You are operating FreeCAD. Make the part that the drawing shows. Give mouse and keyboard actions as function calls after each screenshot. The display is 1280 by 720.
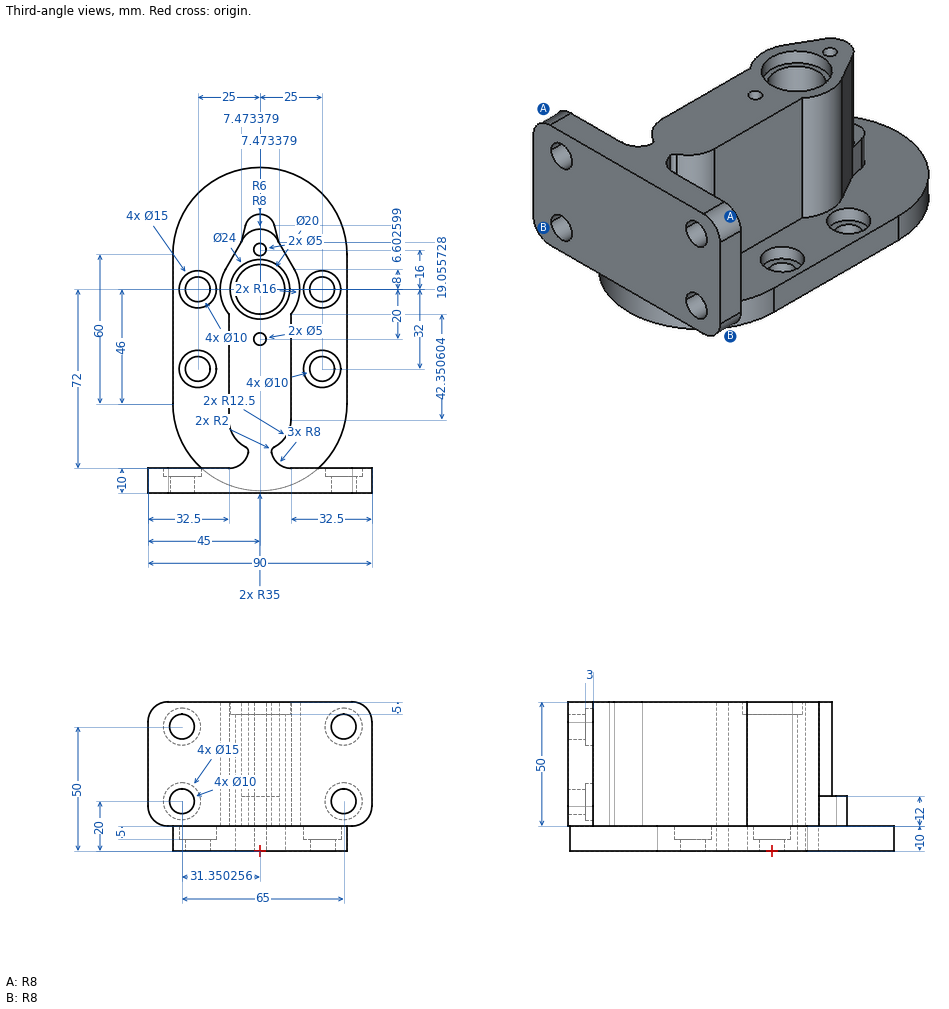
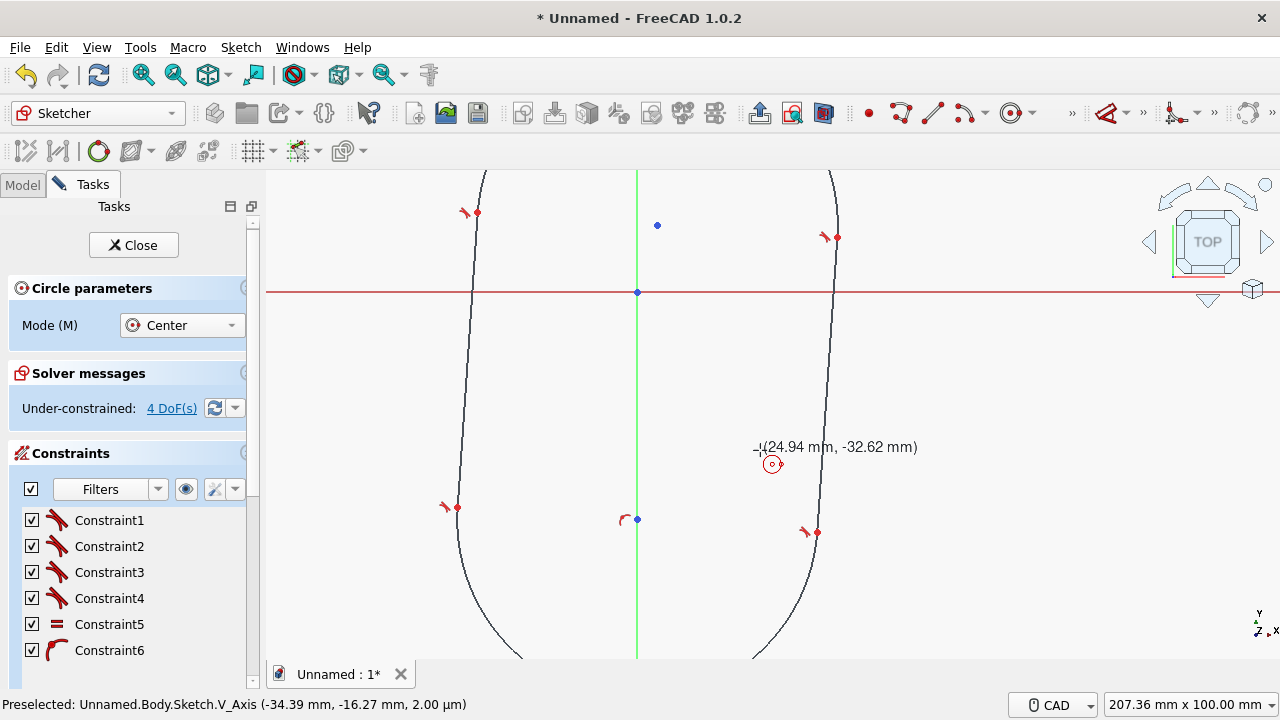
click(760, 448)
click(777, 431)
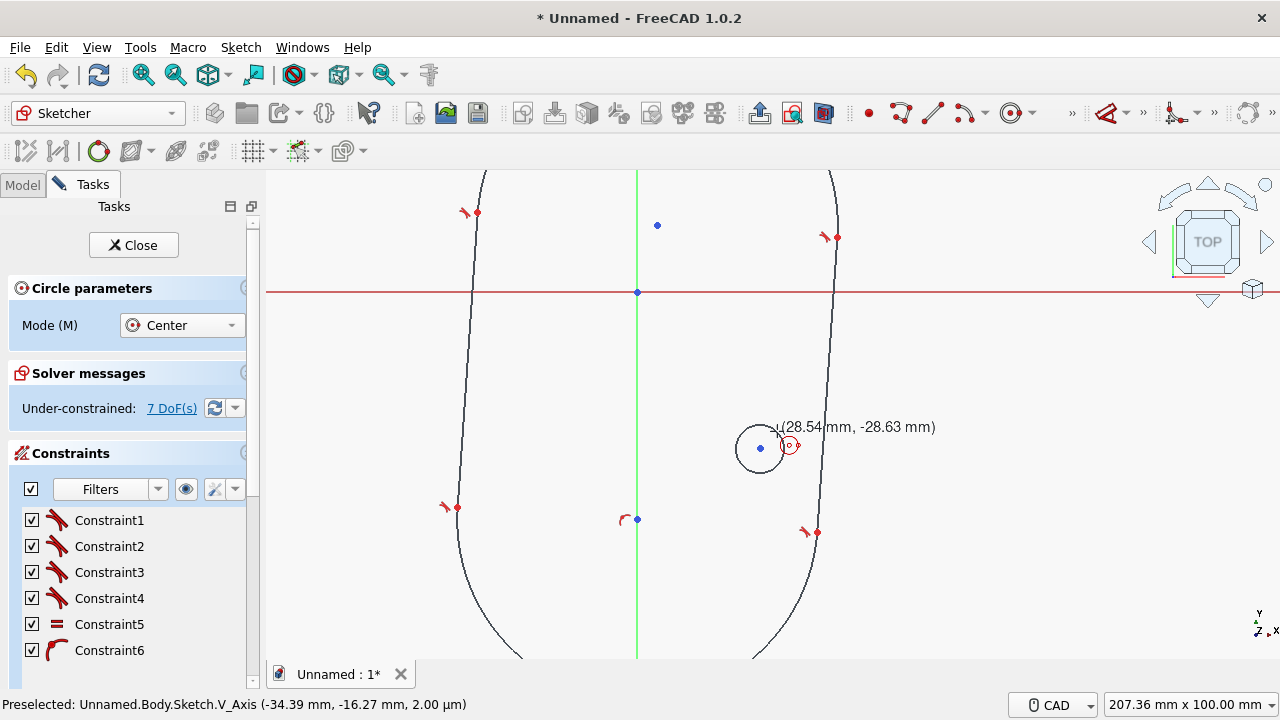
click(515, 448)
click(532, 431)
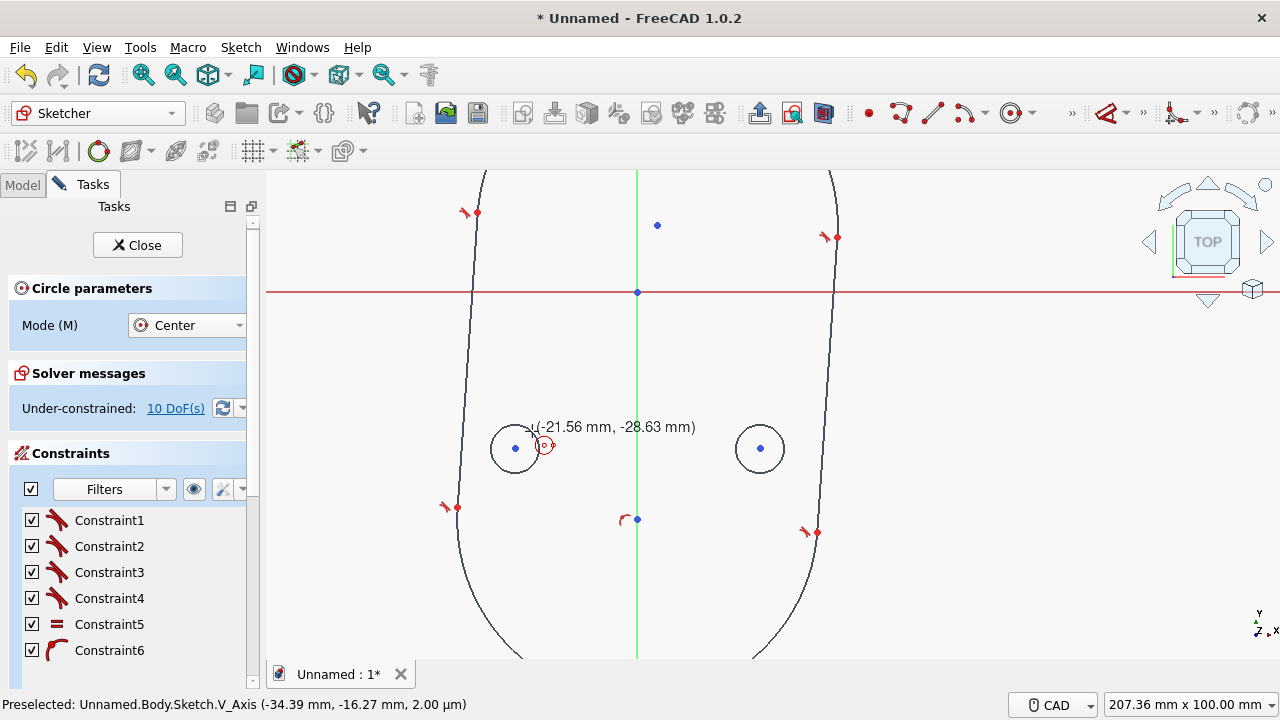
click(760, 292)
click(777, 275)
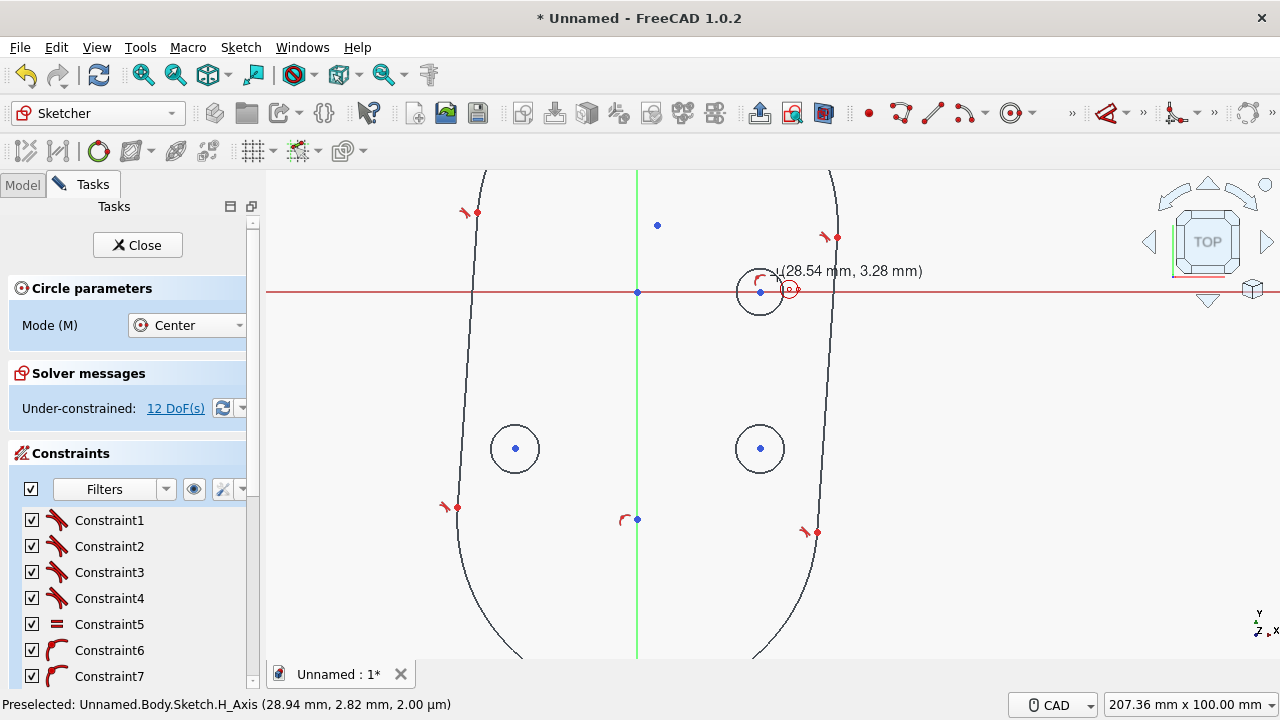
click(515, 292)
click(532, 275)
key(Escape)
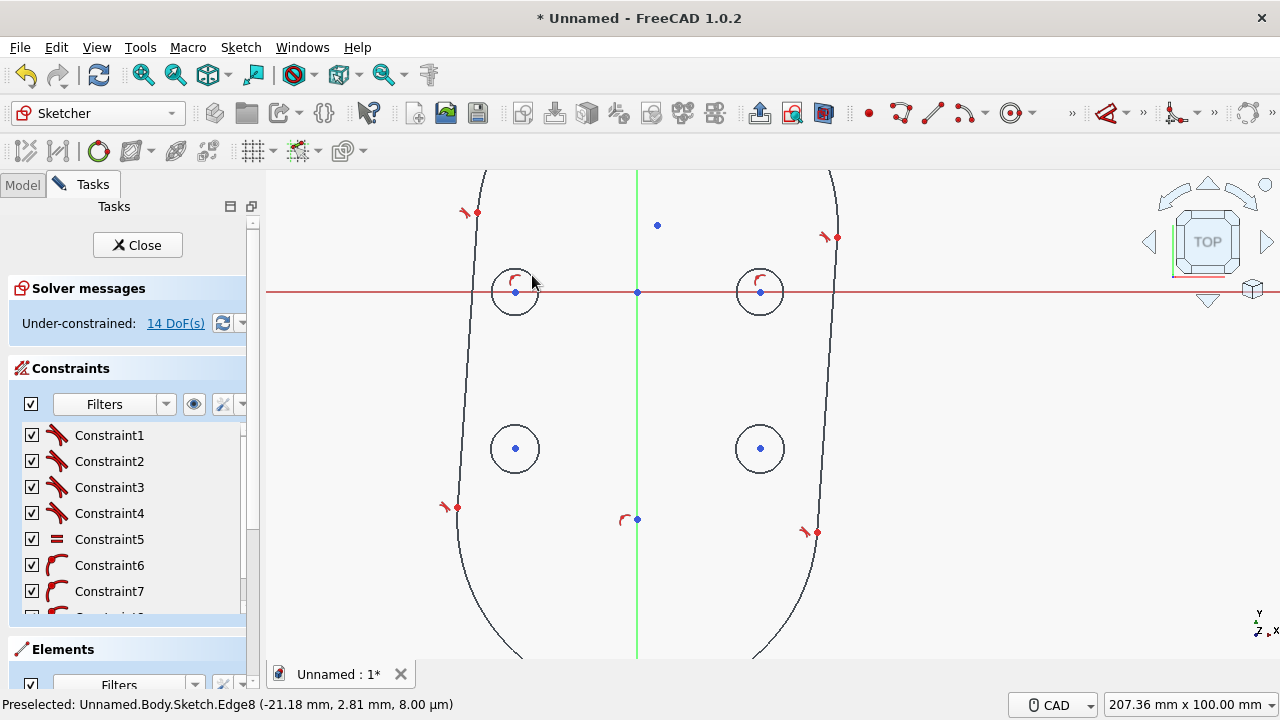
click(464, 419)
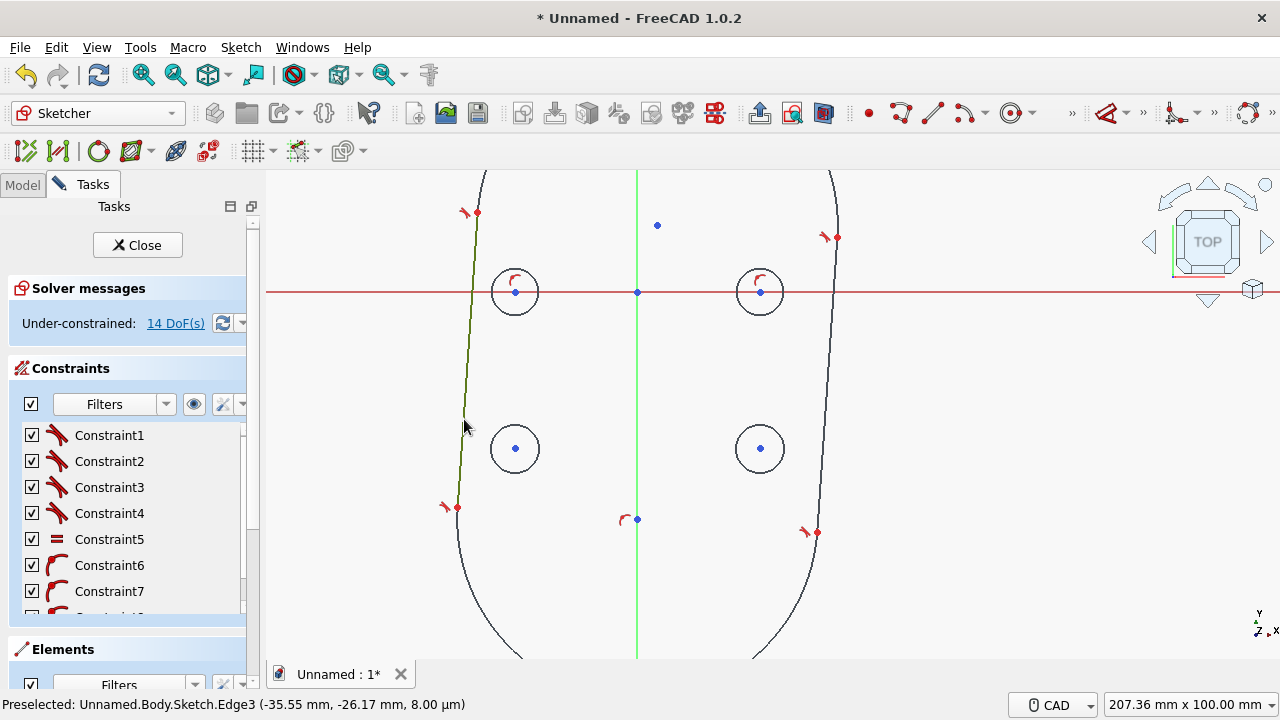
key(v)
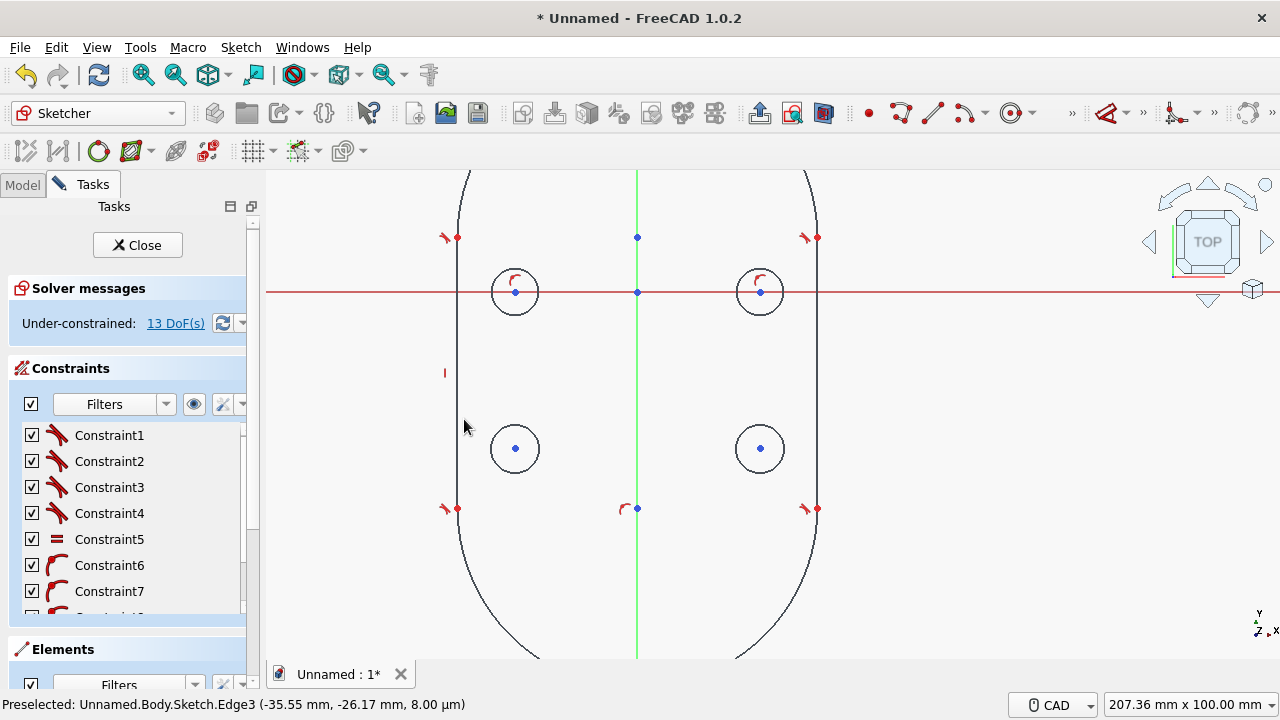
click(777, 432)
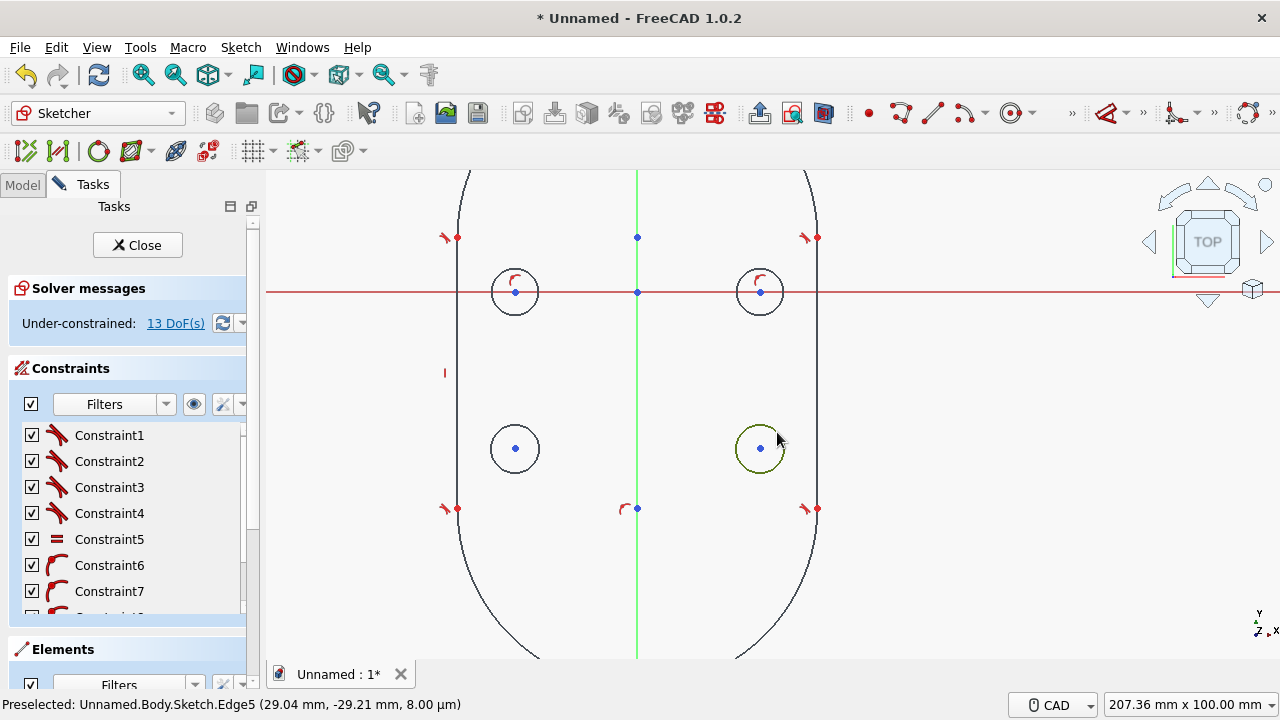
click(532, 432)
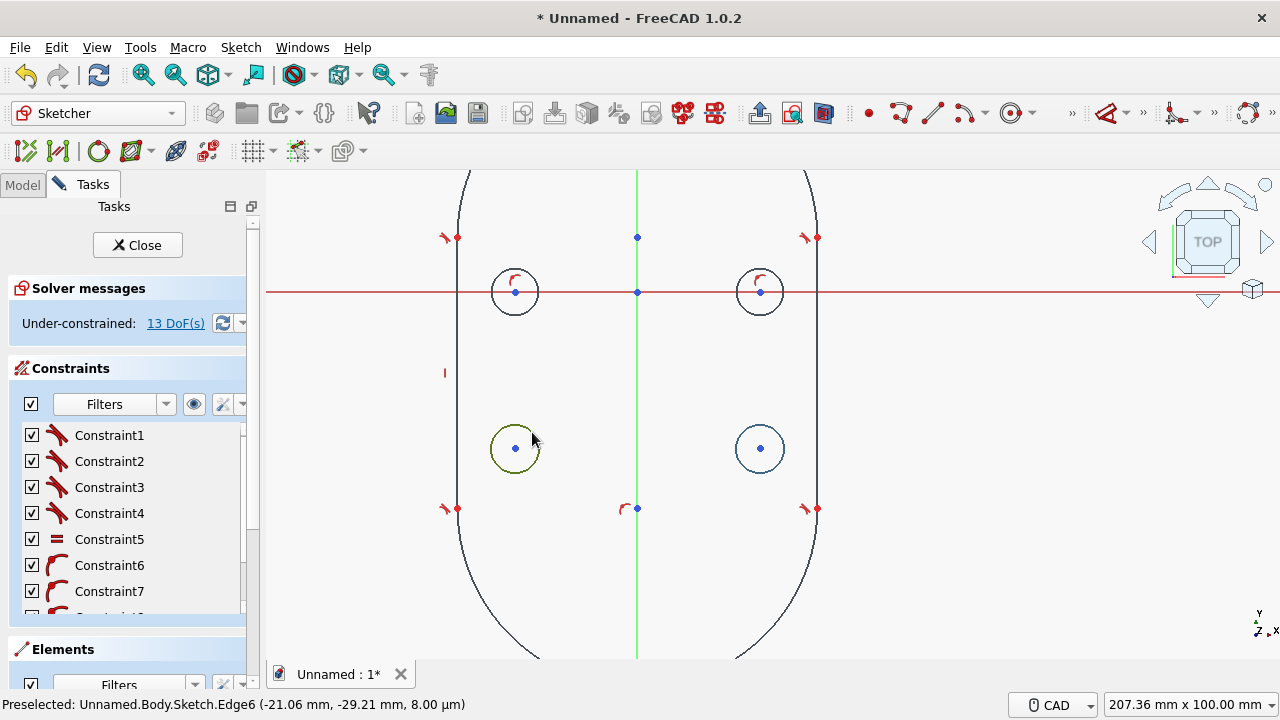
click(776, 275)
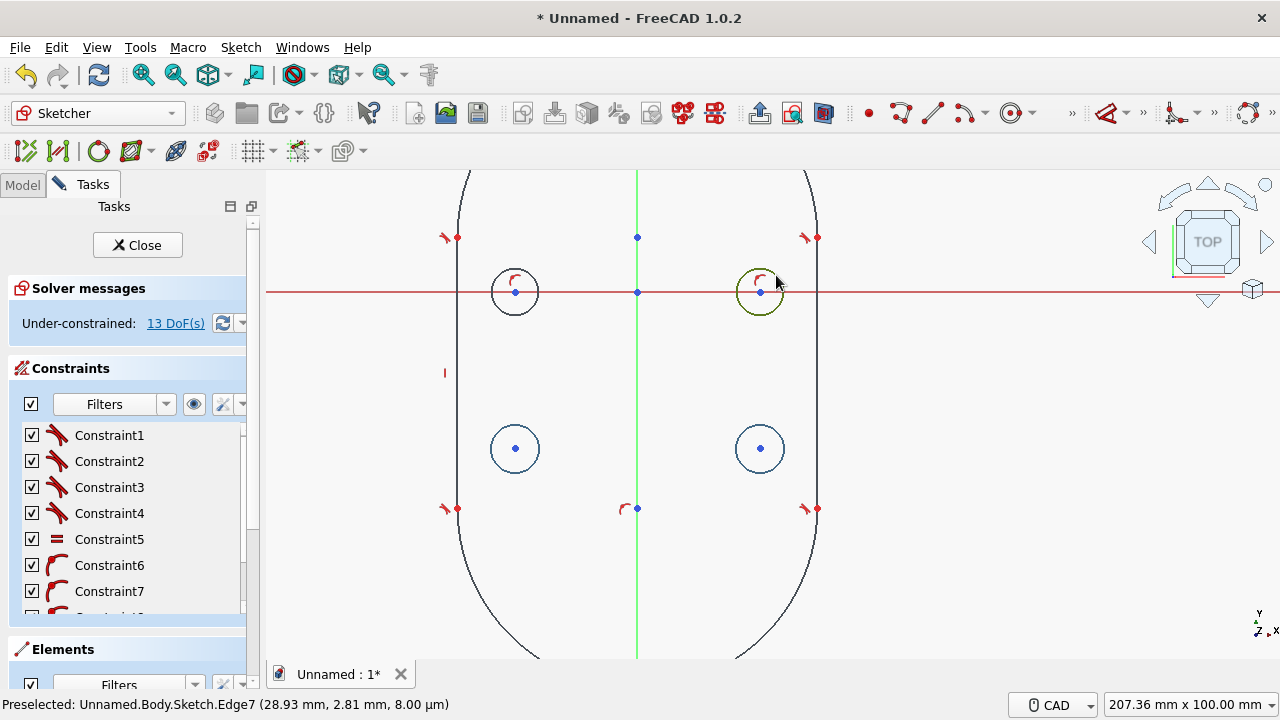
click(531, 275)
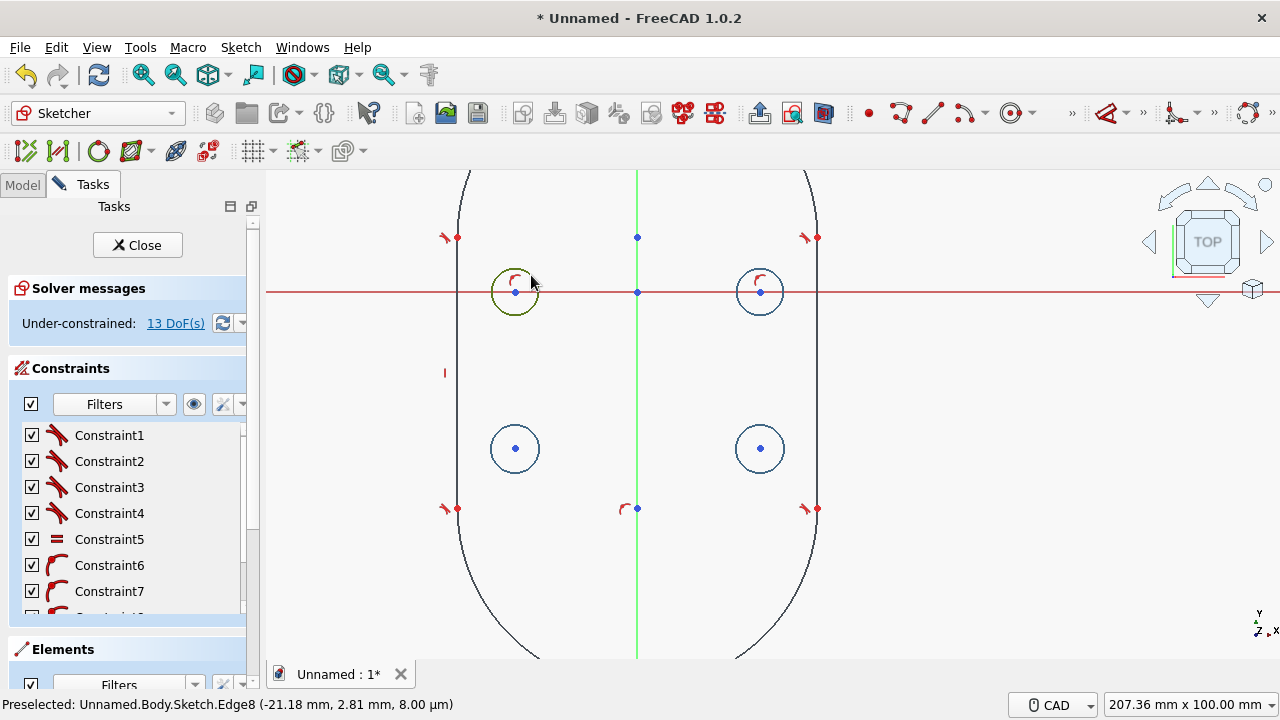
key(e)